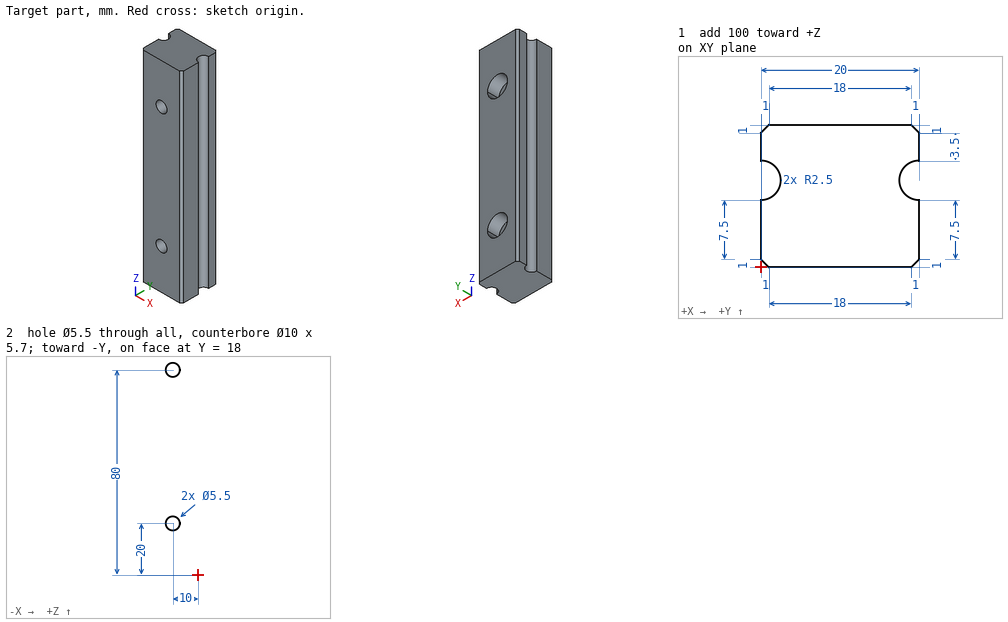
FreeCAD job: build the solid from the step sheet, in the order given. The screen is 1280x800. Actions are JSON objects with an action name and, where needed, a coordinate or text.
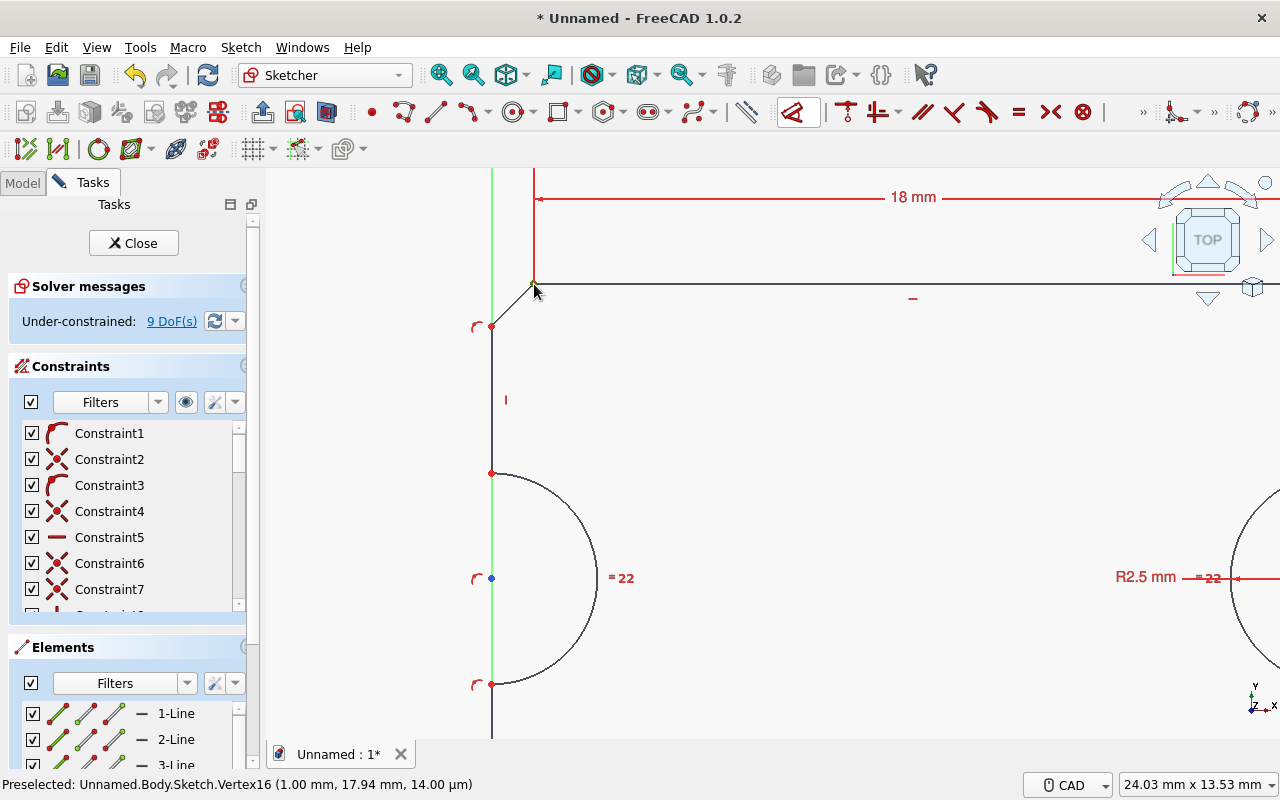
{"action": "key", "text": "l"}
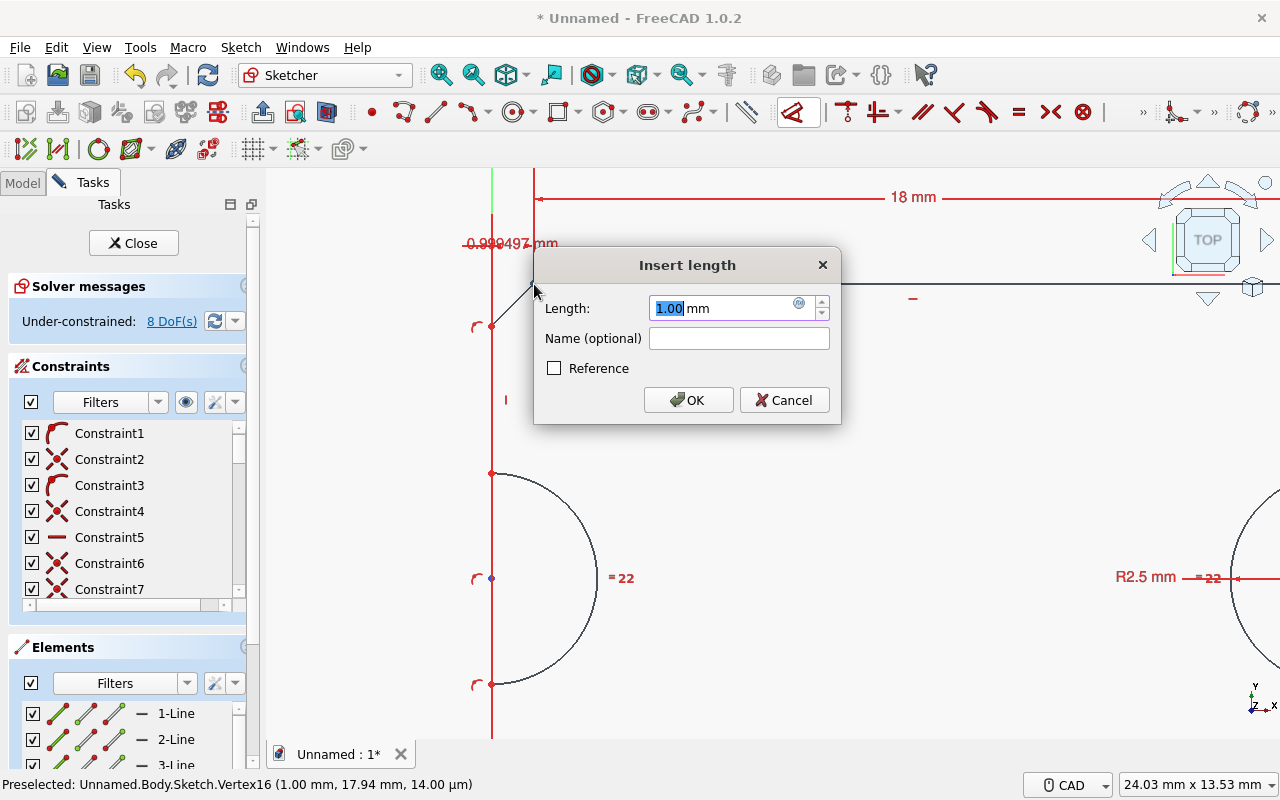
{"action": "type", "text": "1"}
{"action": "key", "text": "Return"}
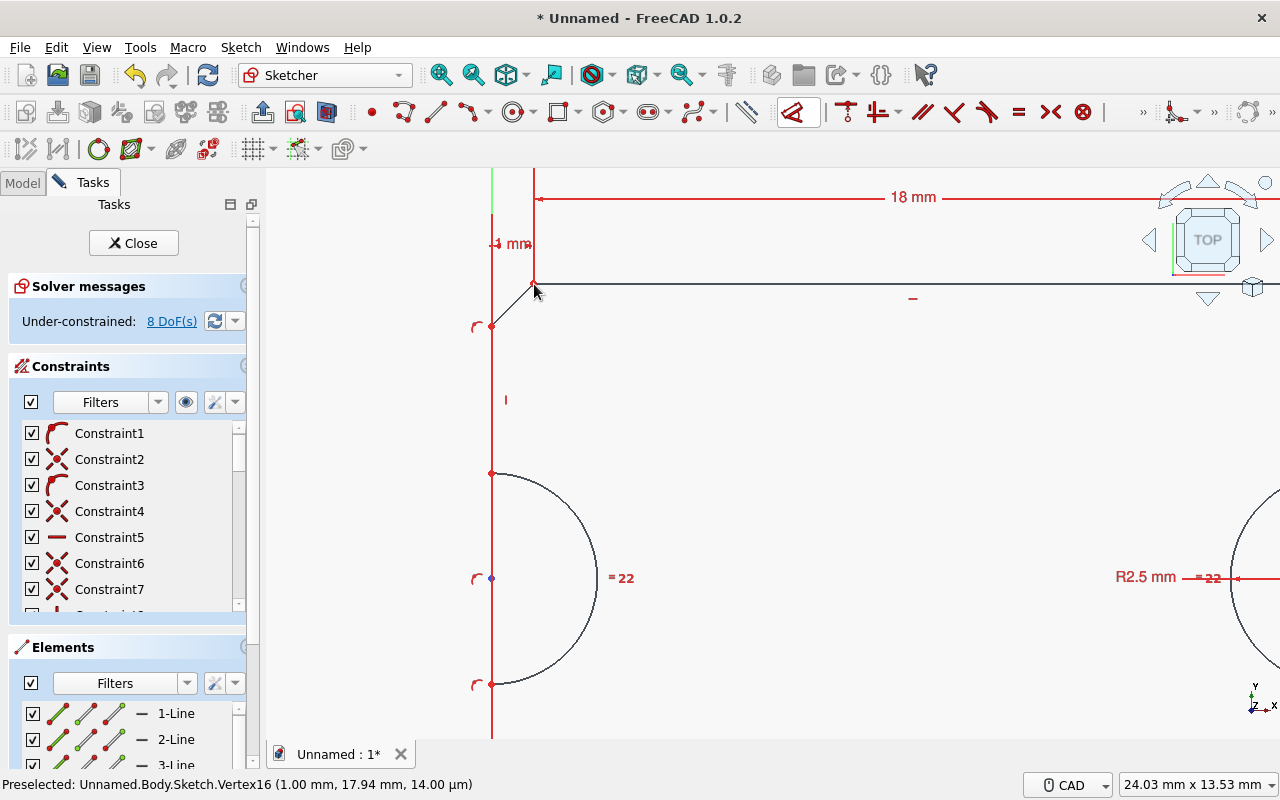
{"action": "scroll", "coordinate": [534, 284], "scroll_direction": "down", "scroll_amount": 4}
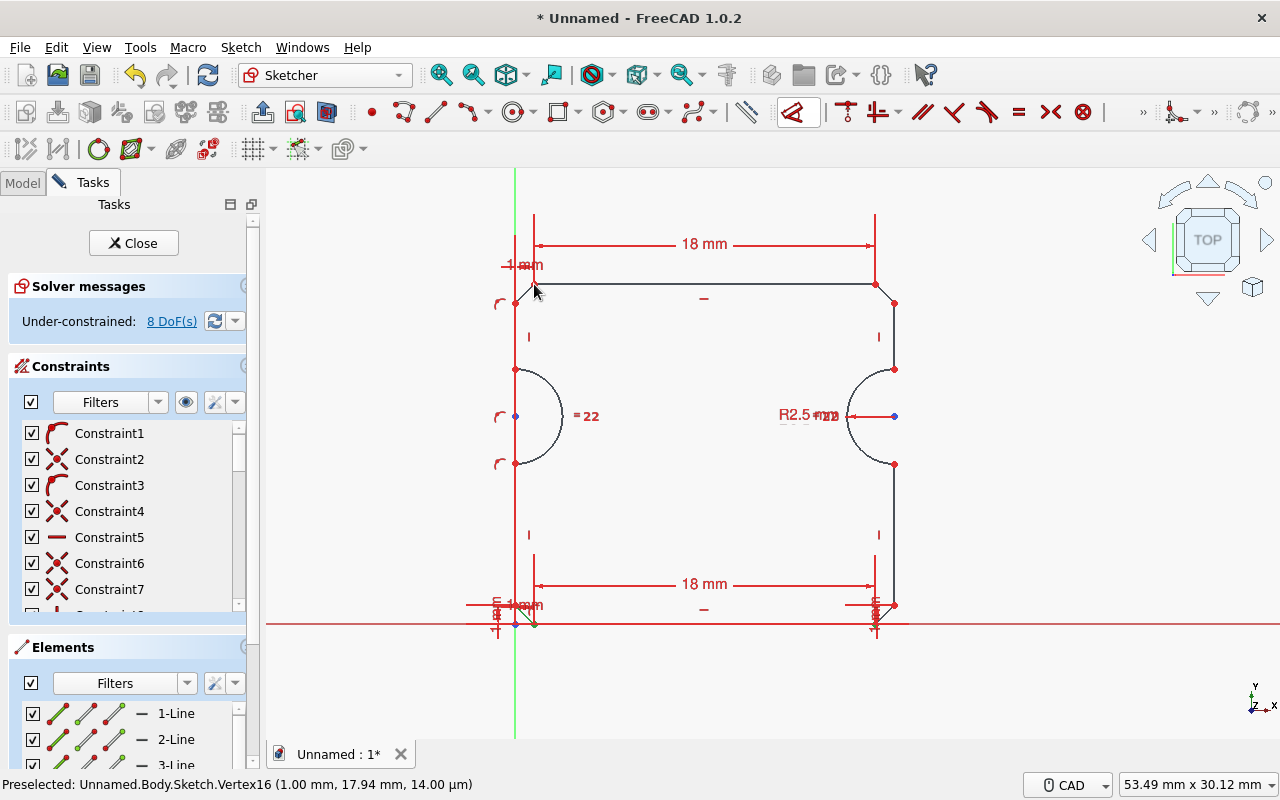
{"action": "scroll", "coordinate": [881, 619], "scroll_direction": "up", "scroll_amount": 5}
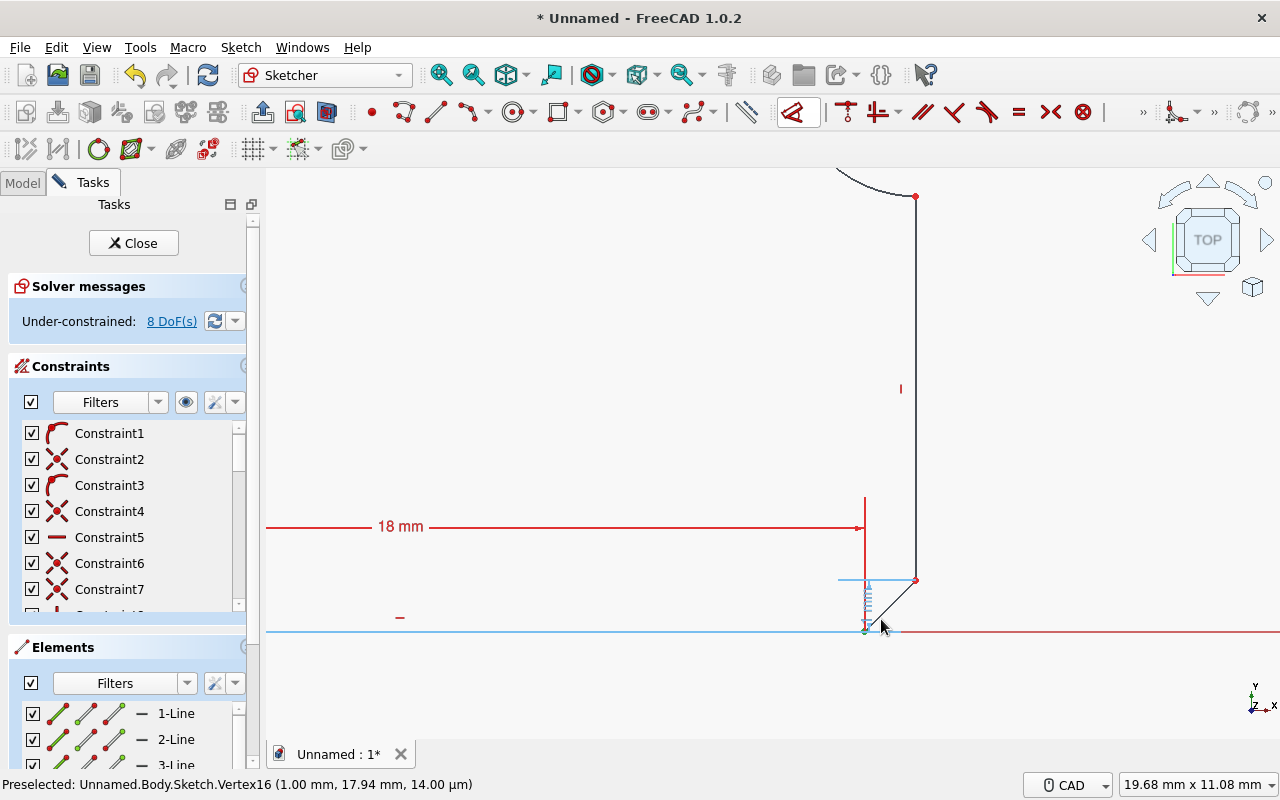
{"action": "left_click", "coordinate": [880, 617]}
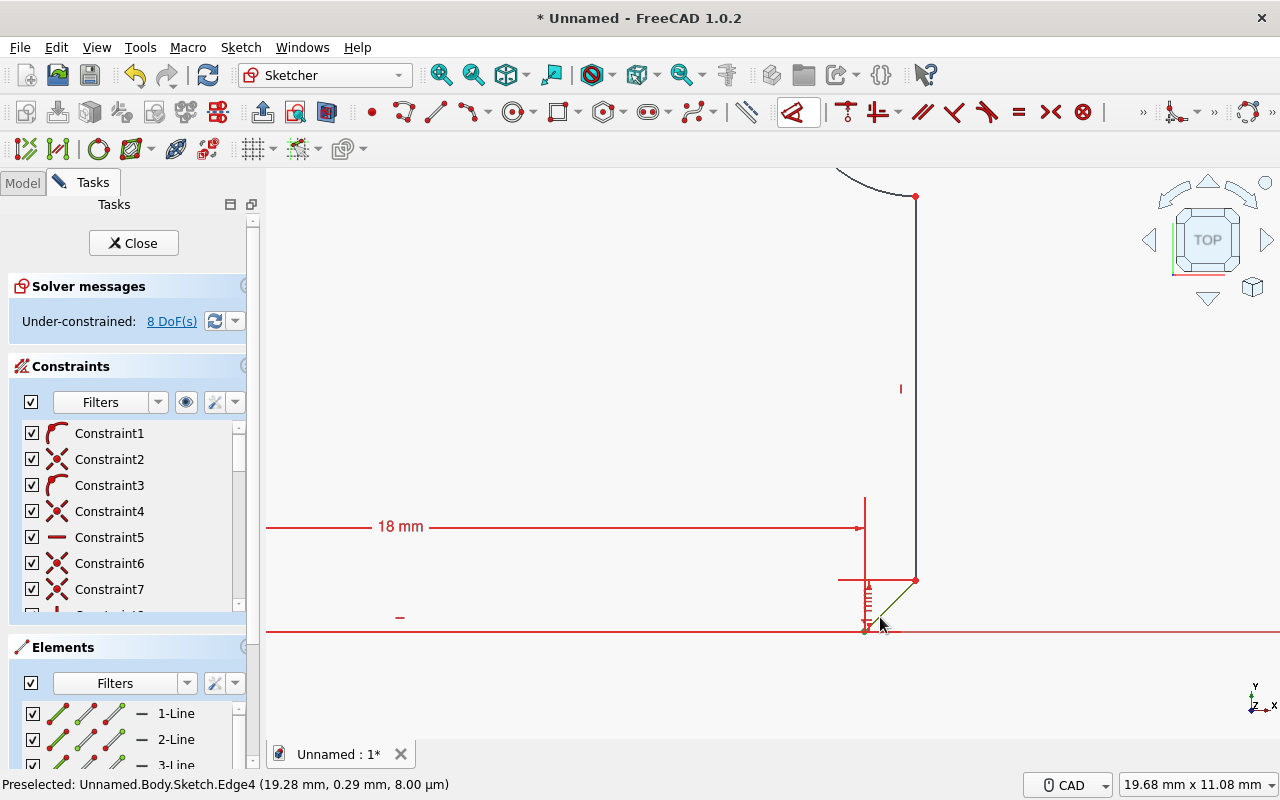
{"action": "key", "text": "l"}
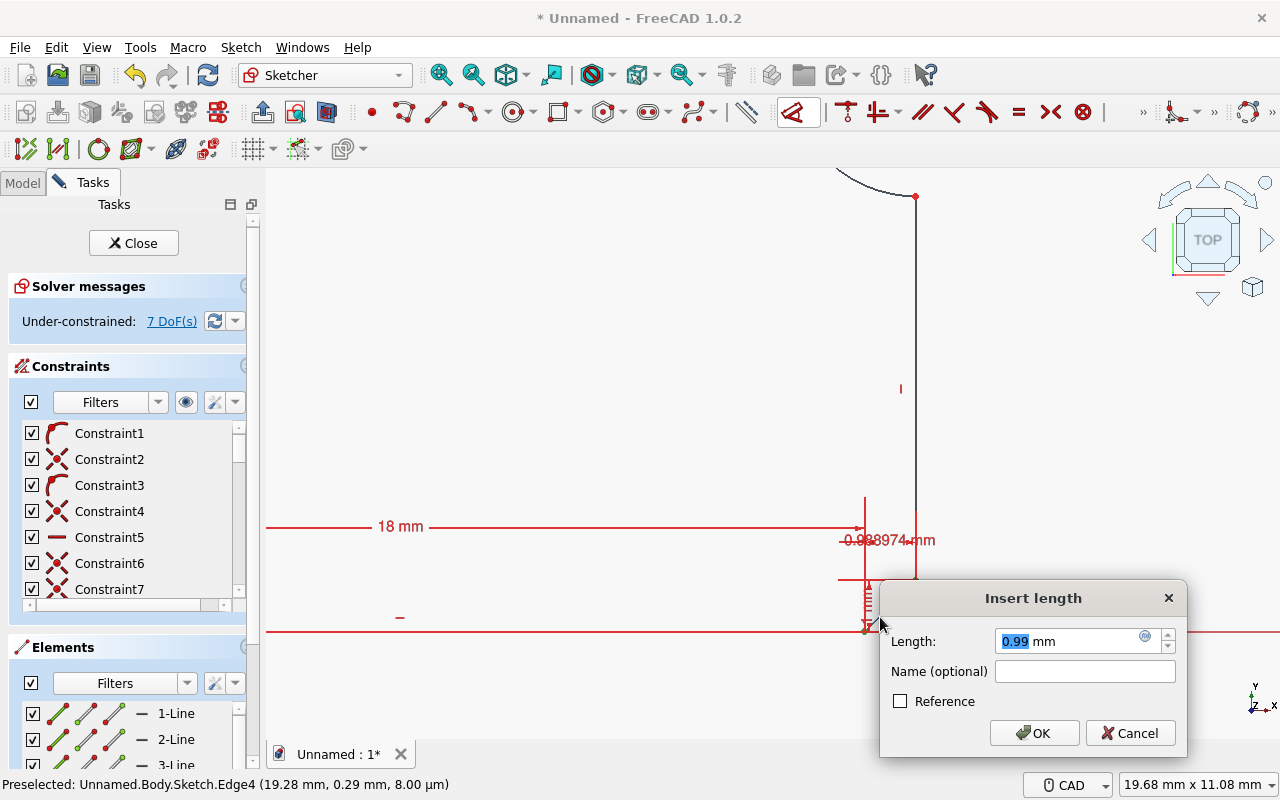
{"action": "type", "text": "1"}
{"action": "key", "text": "Return"}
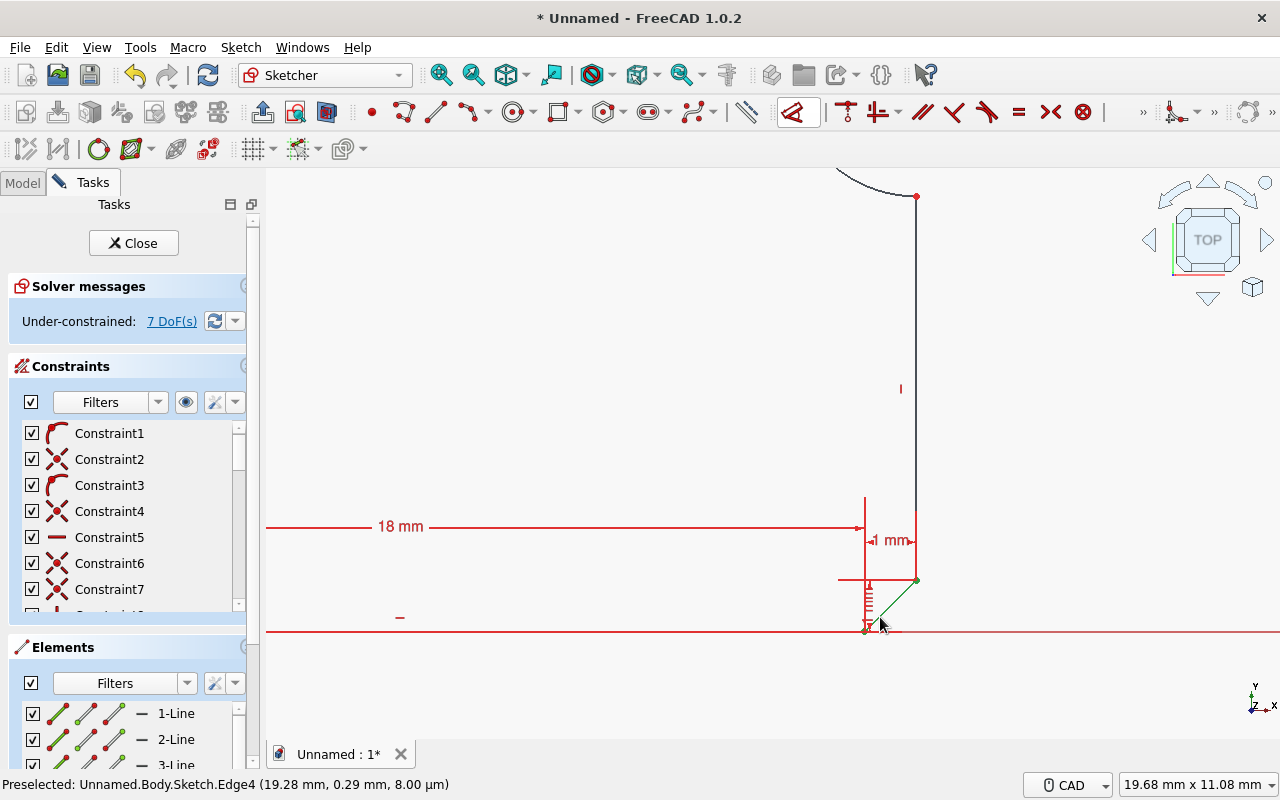
{"action": "scroll", "coordinate": [881, 620], "scroll_direction": "down", "scroll_amount": 5}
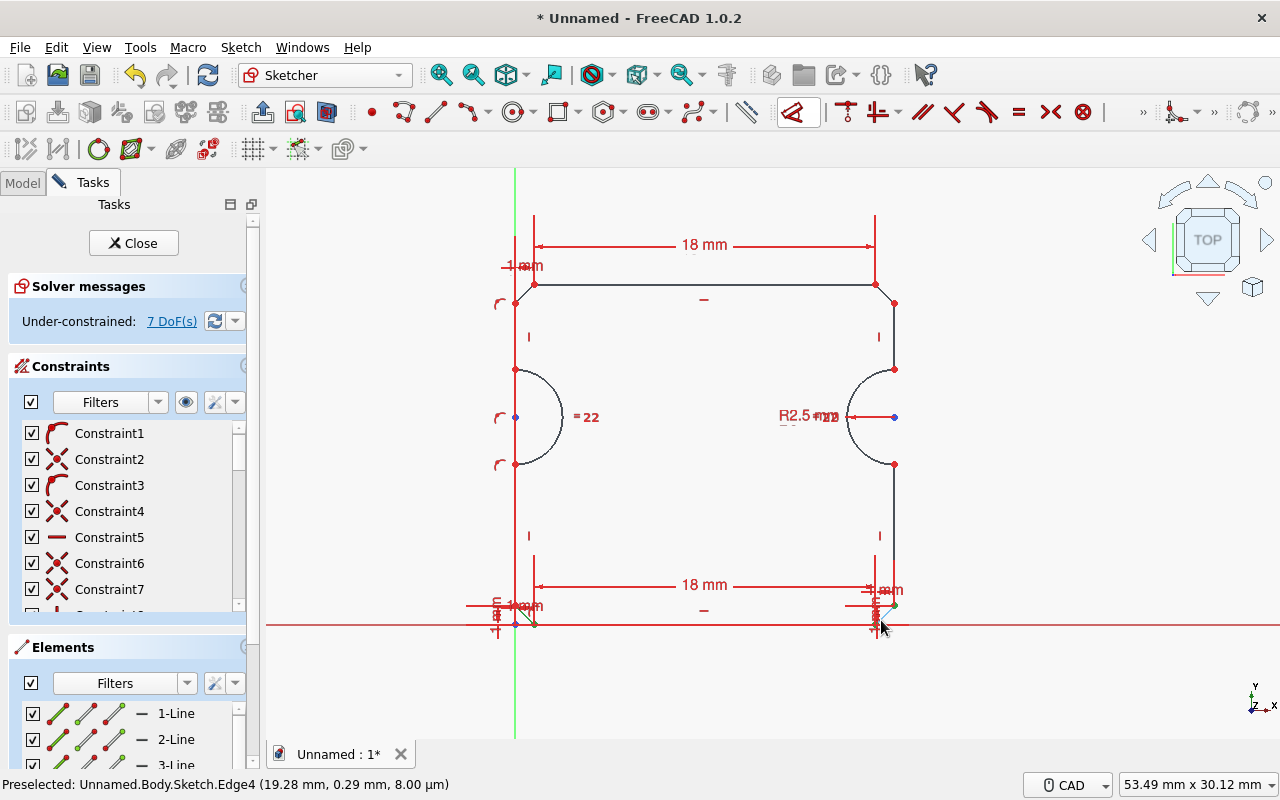
{"action": "scroll", "coordinate": [888, 298], "scroll_direction": "up", "scroll_amount": 4}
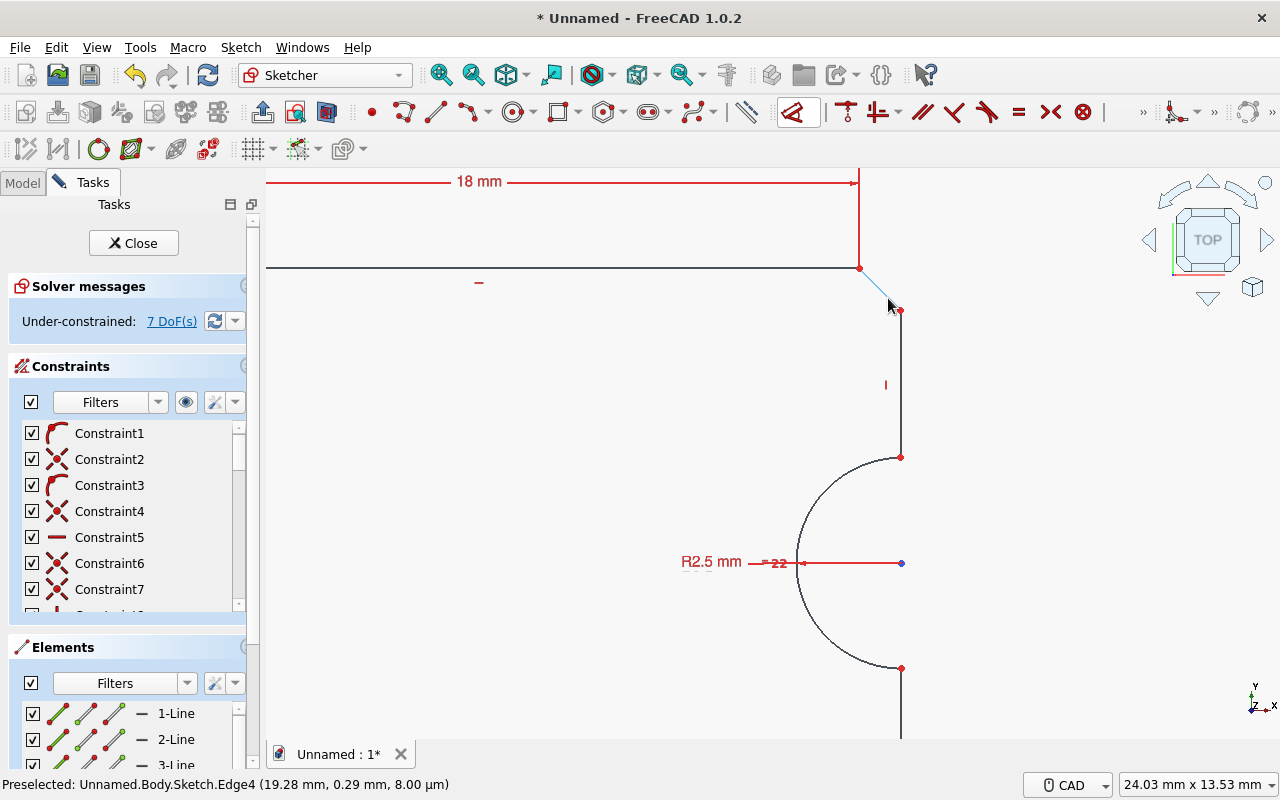
{"action": "left_click", "coordinate": [888, 298]}